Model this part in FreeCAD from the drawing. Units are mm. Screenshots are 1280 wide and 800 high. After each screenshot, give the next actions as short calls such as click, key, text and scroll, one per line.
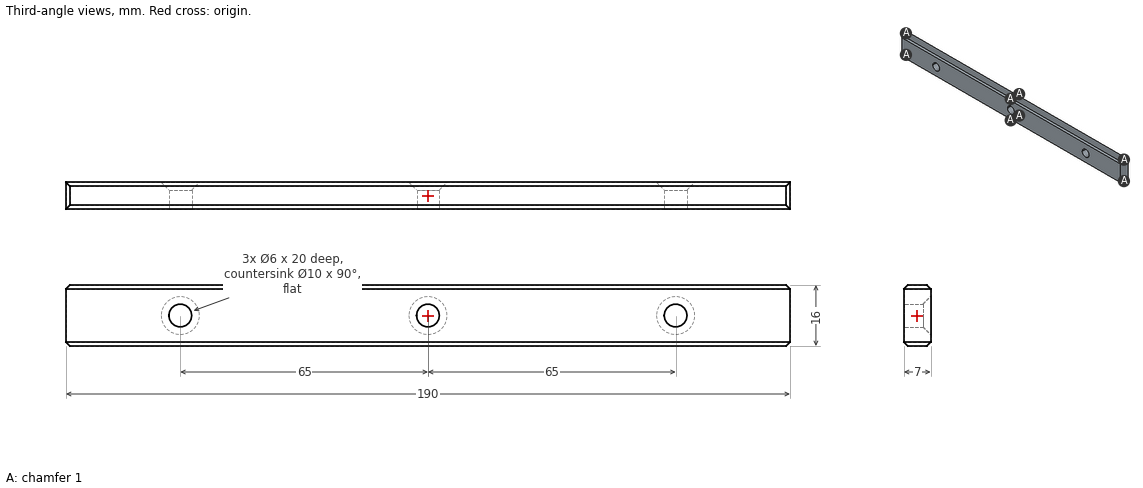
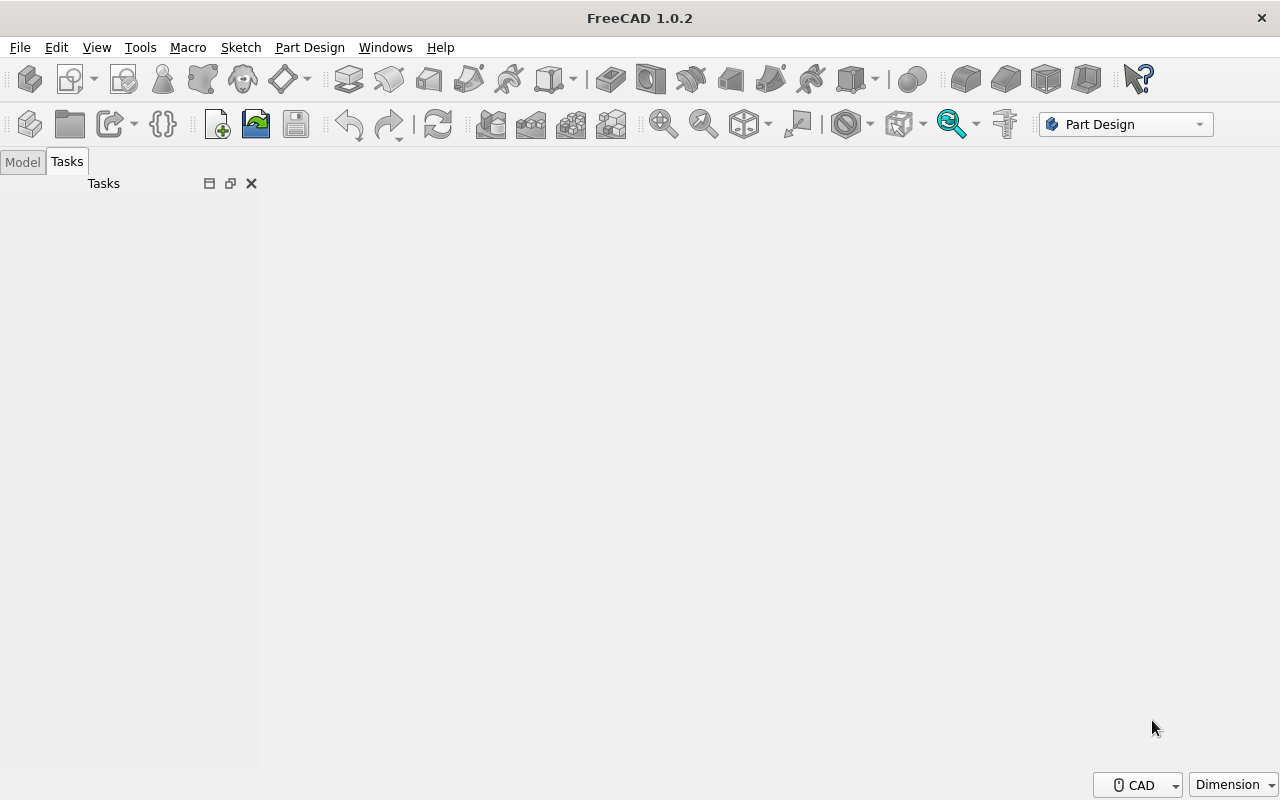
click(216, 124)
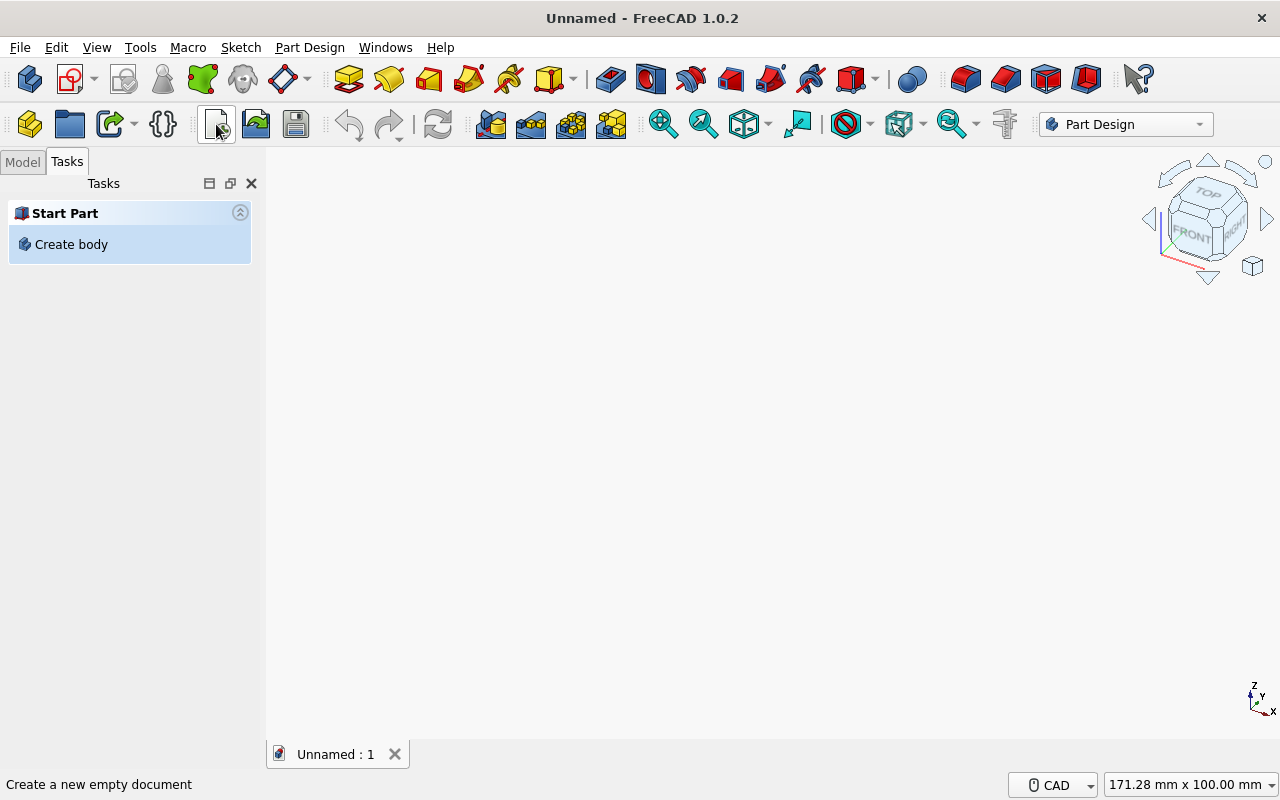
click(70, 80)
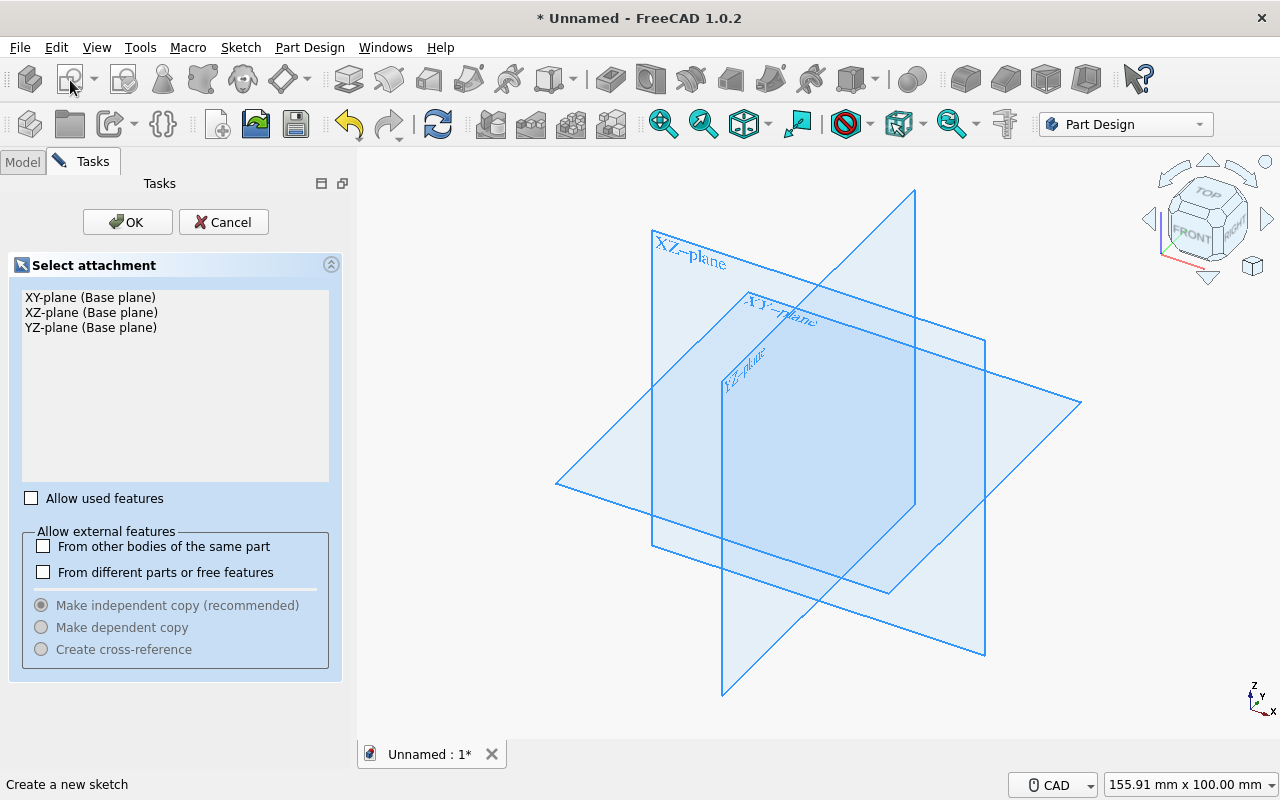
click(82, 312)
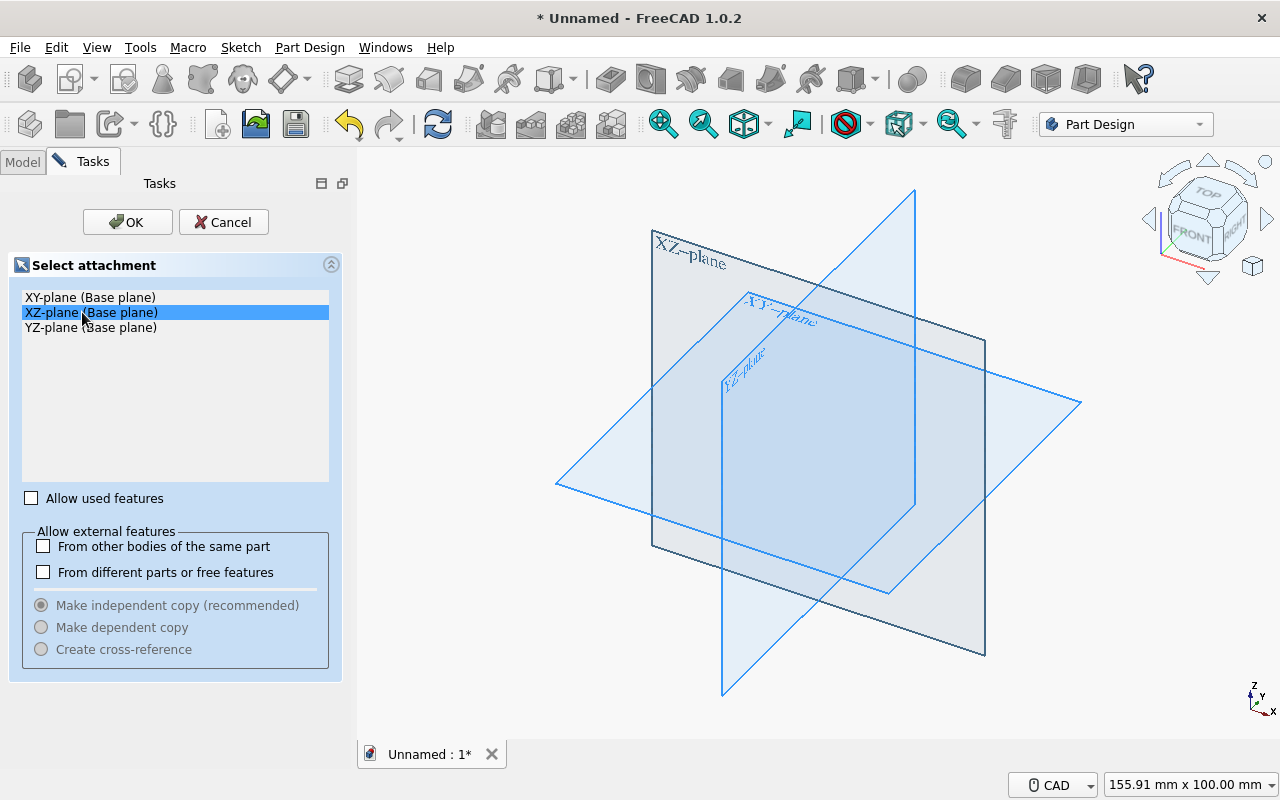
click(128, 222)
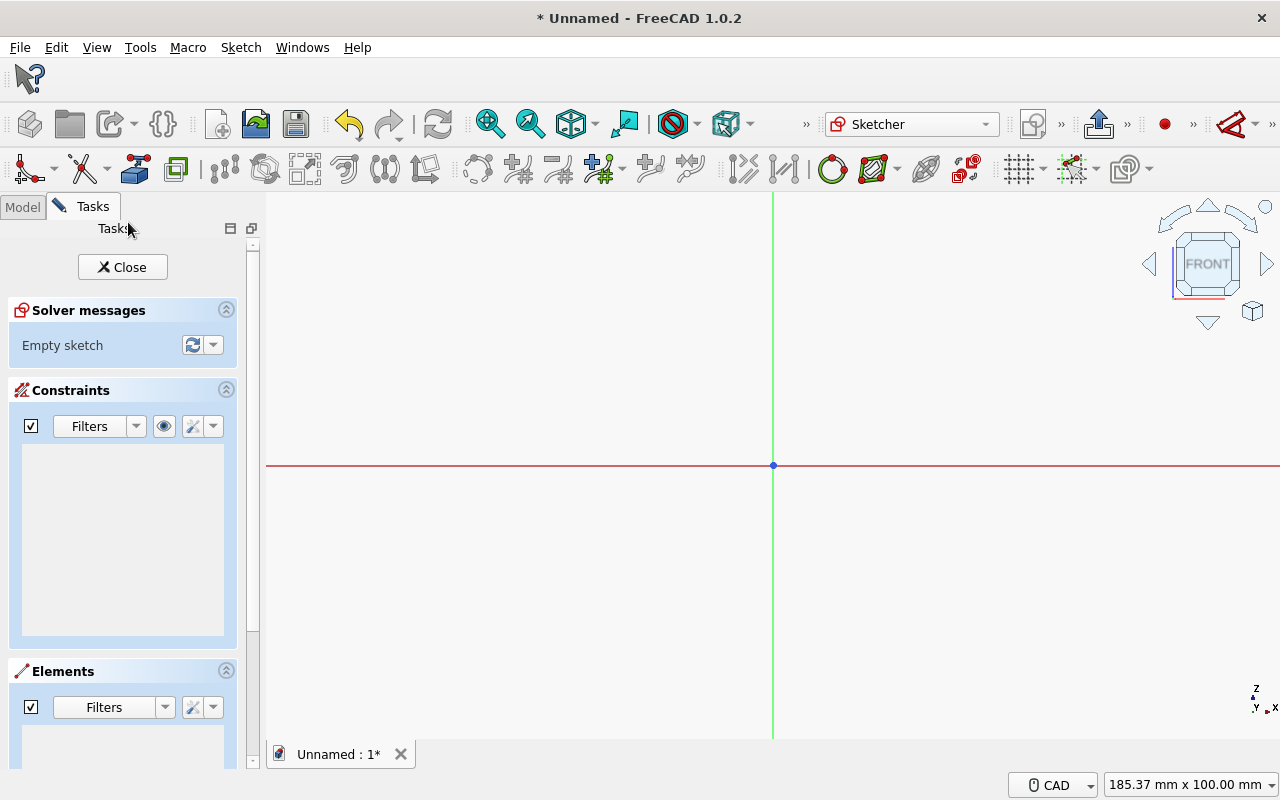
scroll(621, 466, down, 3)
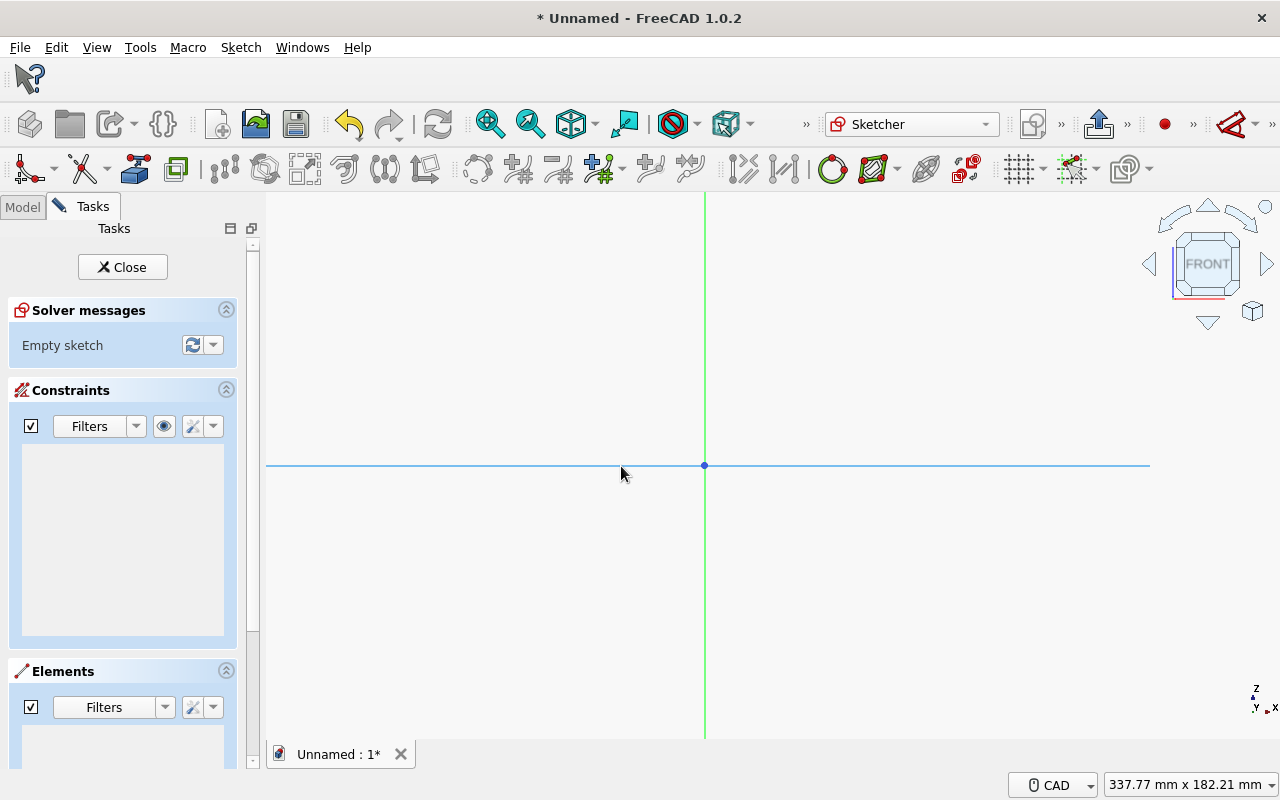
key(g)
key(v)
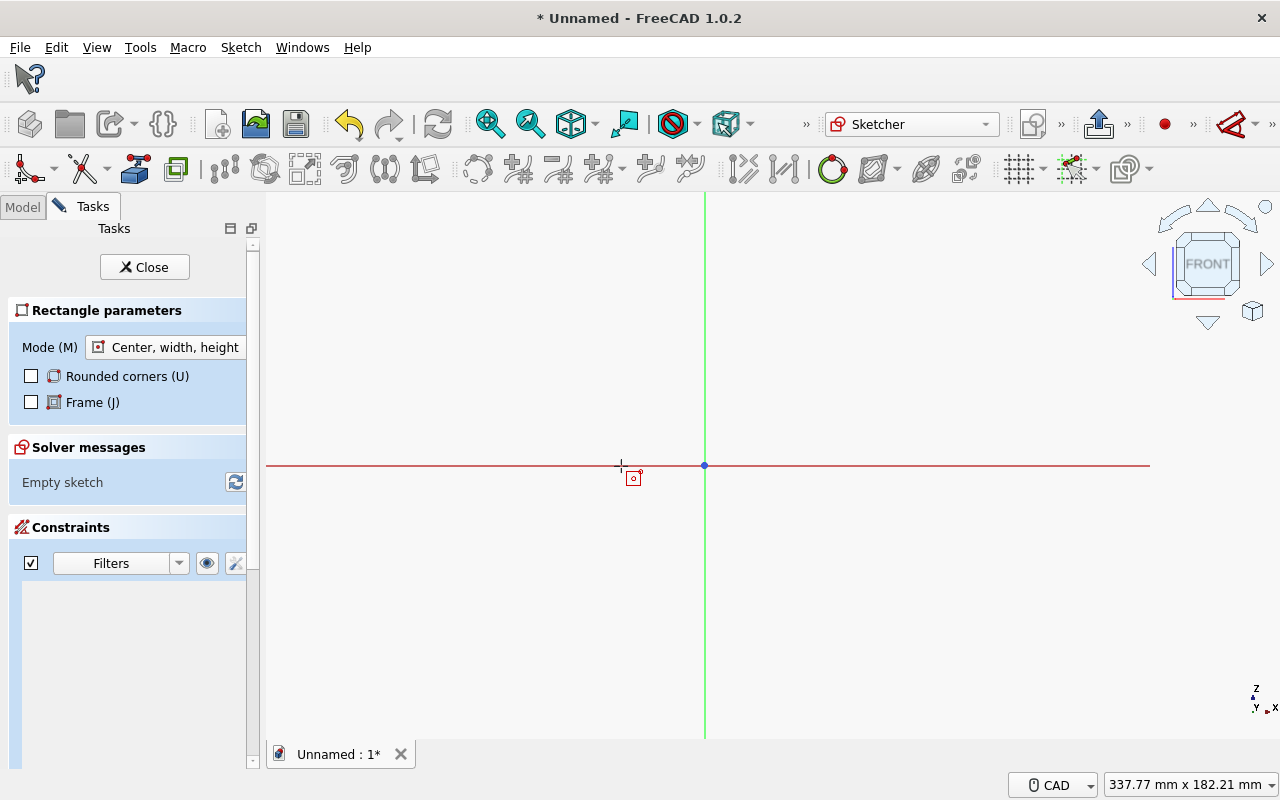
click(705, 466)
click(990, 442)
key(Escape)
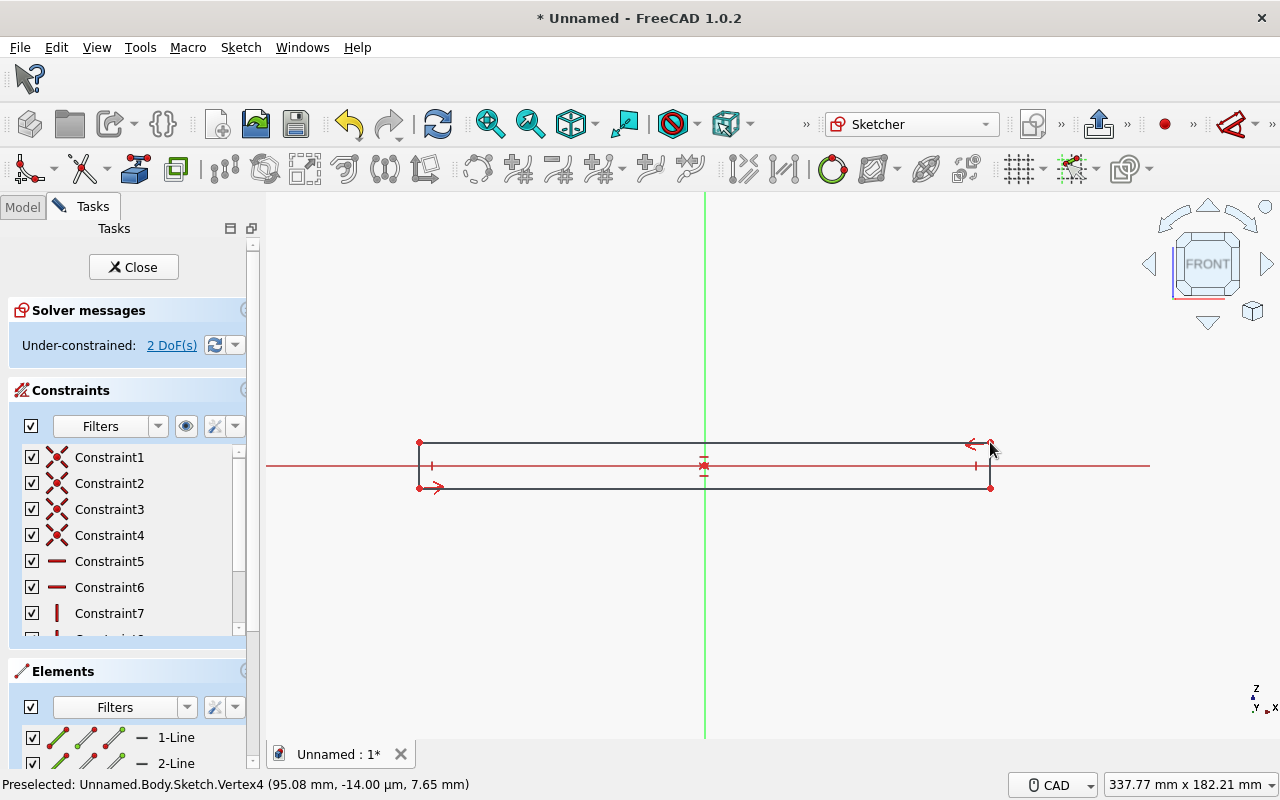
click(1232, 124)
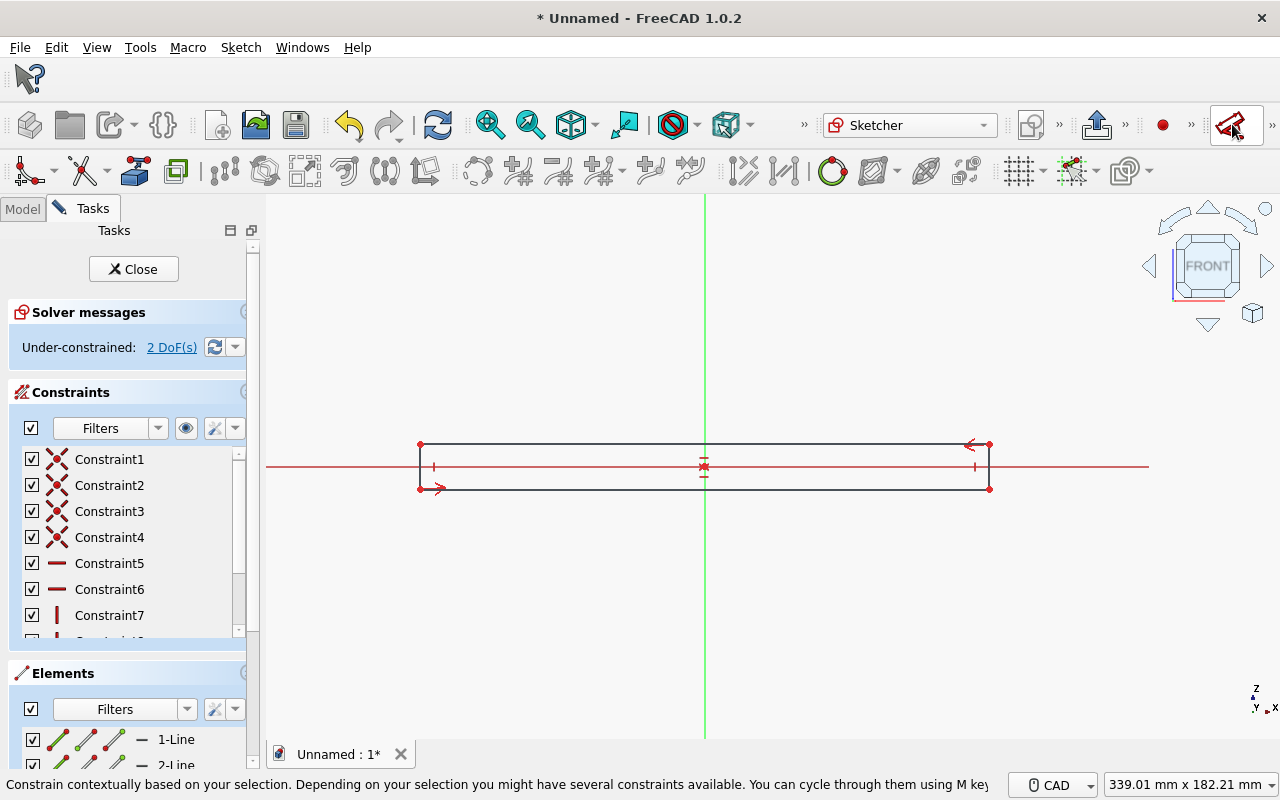
scroll(989, 476, up, 3)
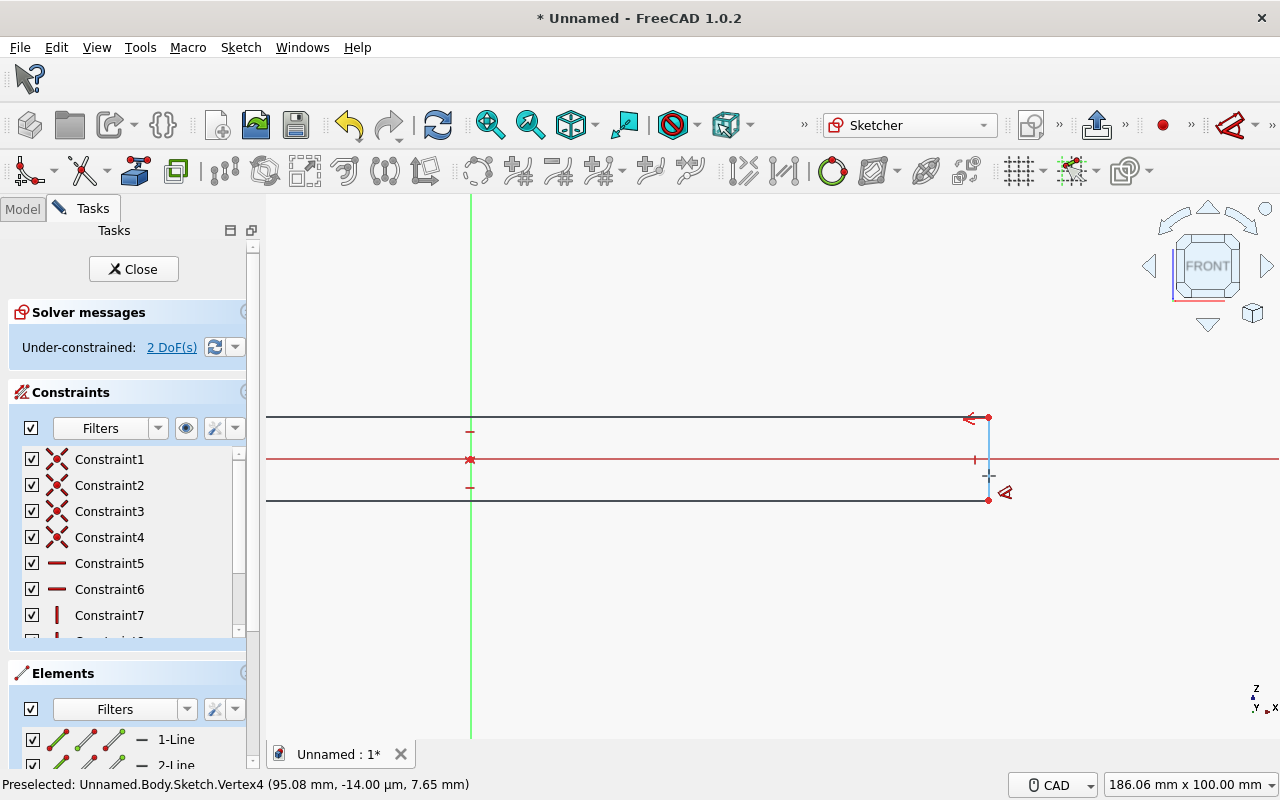
click(989, 476)
click(1023, 440)